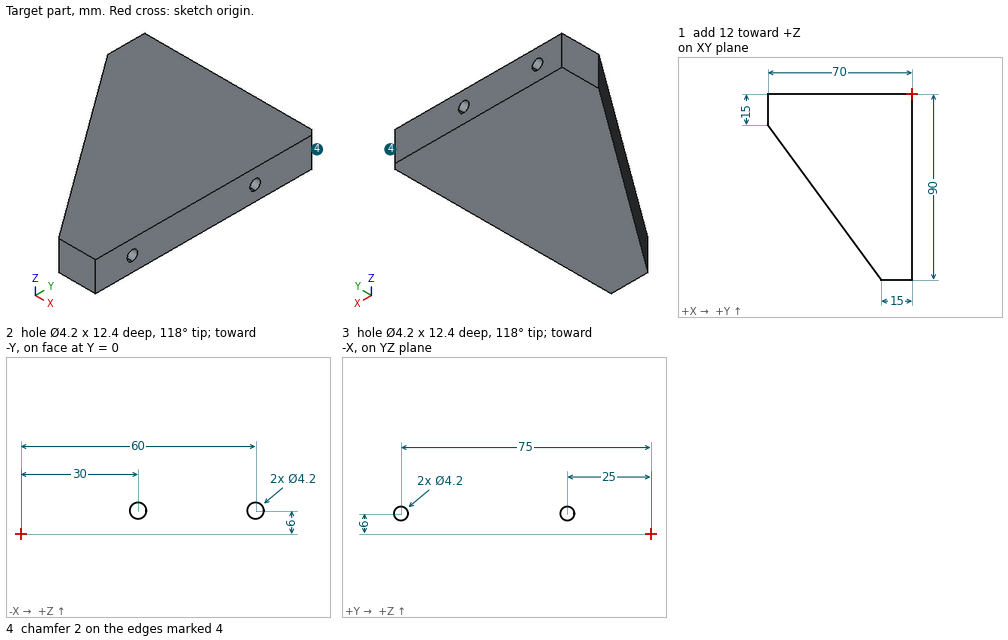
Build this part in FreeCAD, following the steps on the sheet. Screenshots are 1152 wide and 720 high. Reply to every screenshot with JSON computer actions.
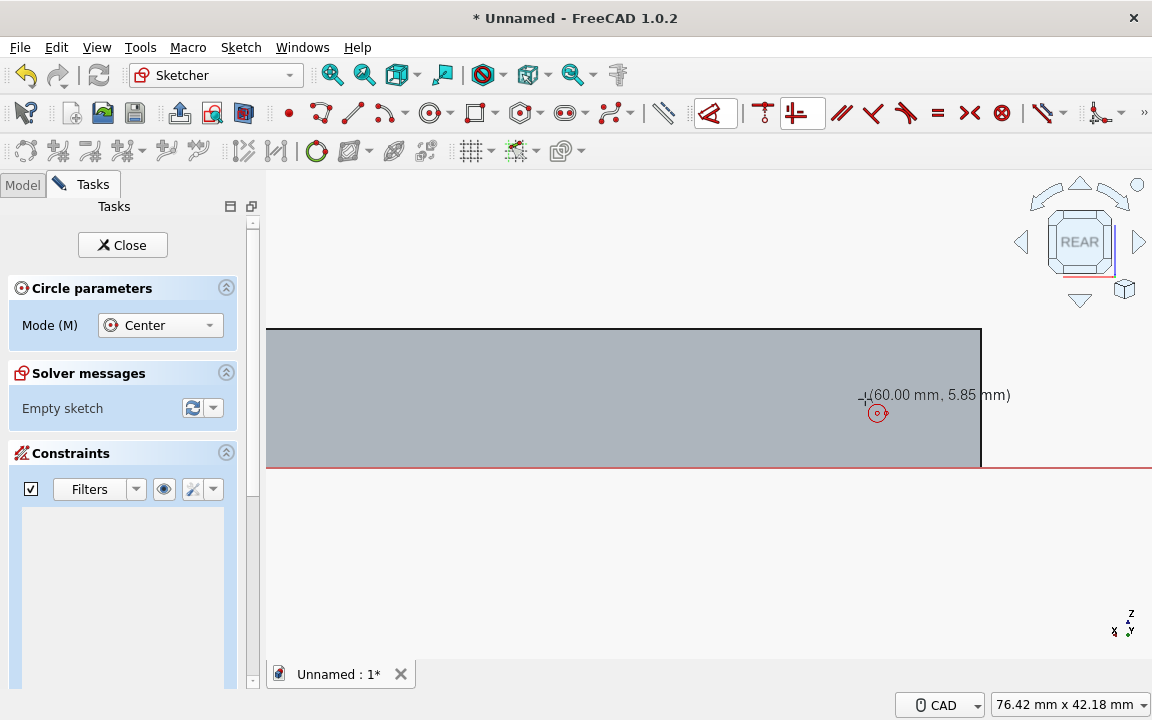
{"action": "left_click", "coordinate": [865, 399]}
{"action": "left_click", "coordinate": [882, 381]}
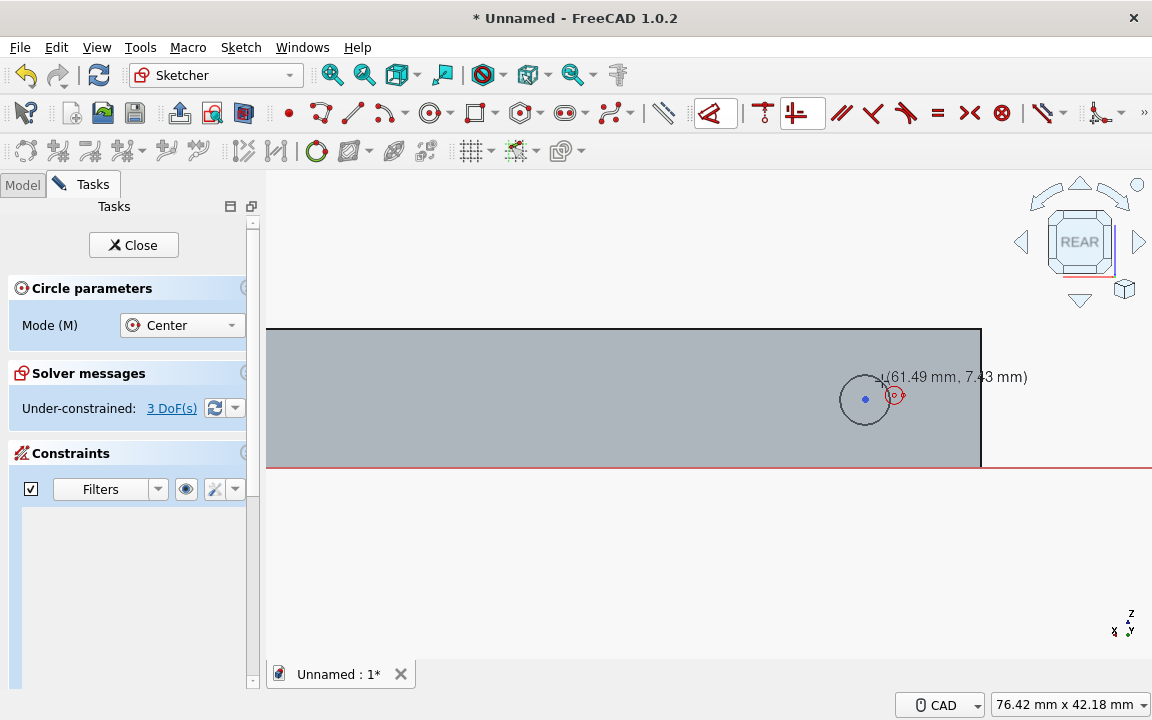
{"action": "left_click", "coordinate": [517, 399]}
{"action": "left_click", "coordinate": [534, 381]}
{"action": "key", "text": "Escape"}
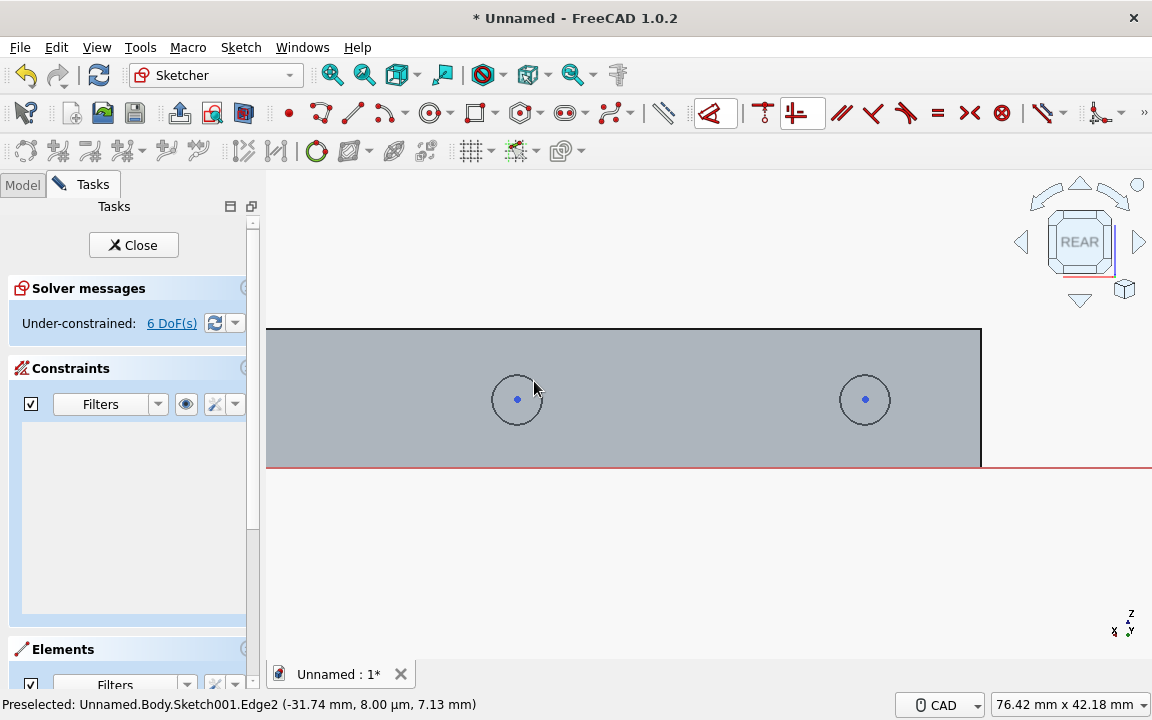
{"action": "left_click", "coordinate": [882, 382]}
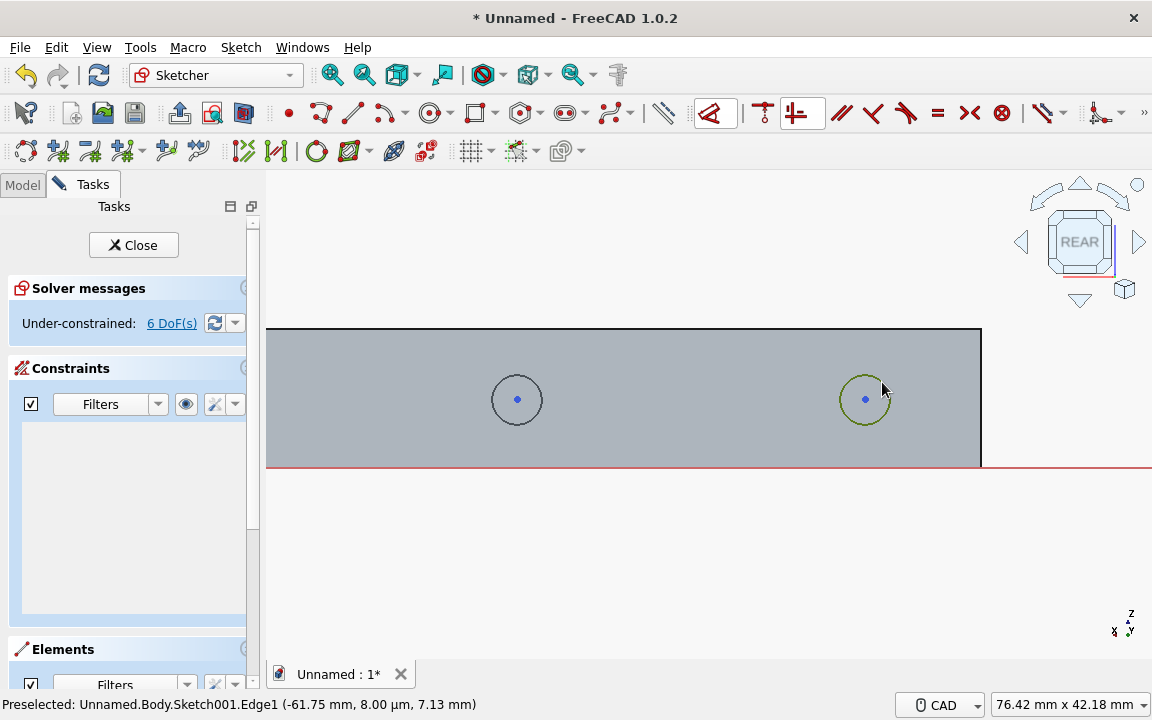
{"action": "left_click", "coordinate": [534, 382]}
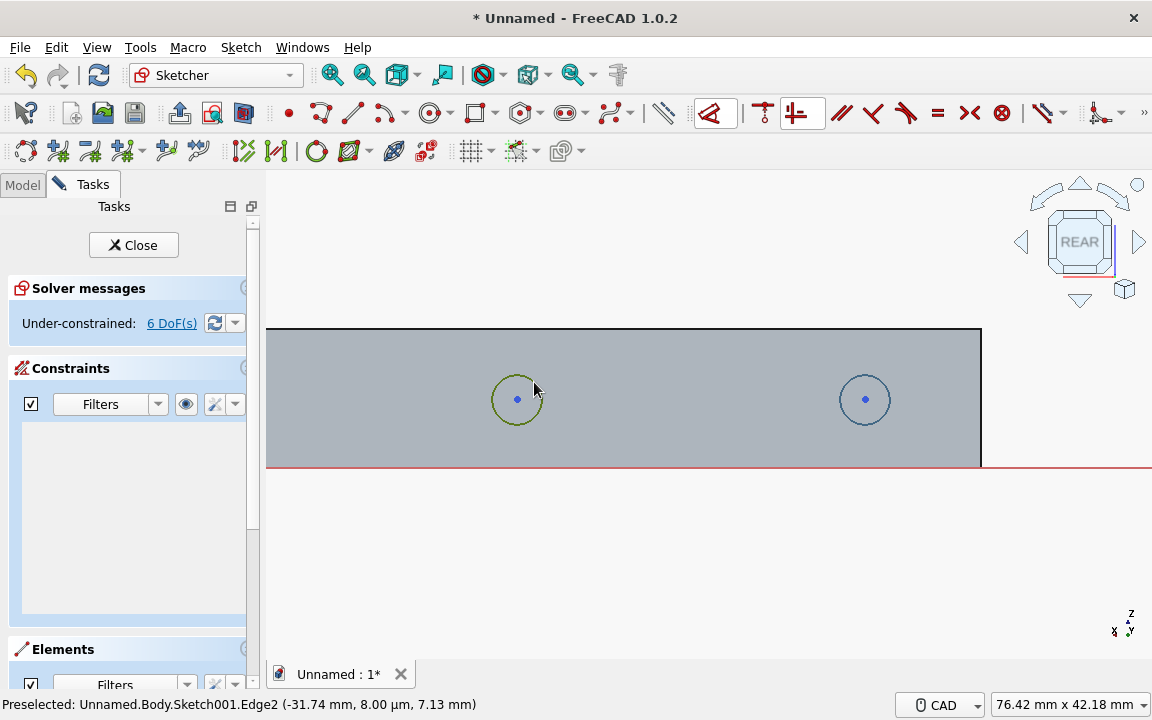
{"action": "key", "text": "e"}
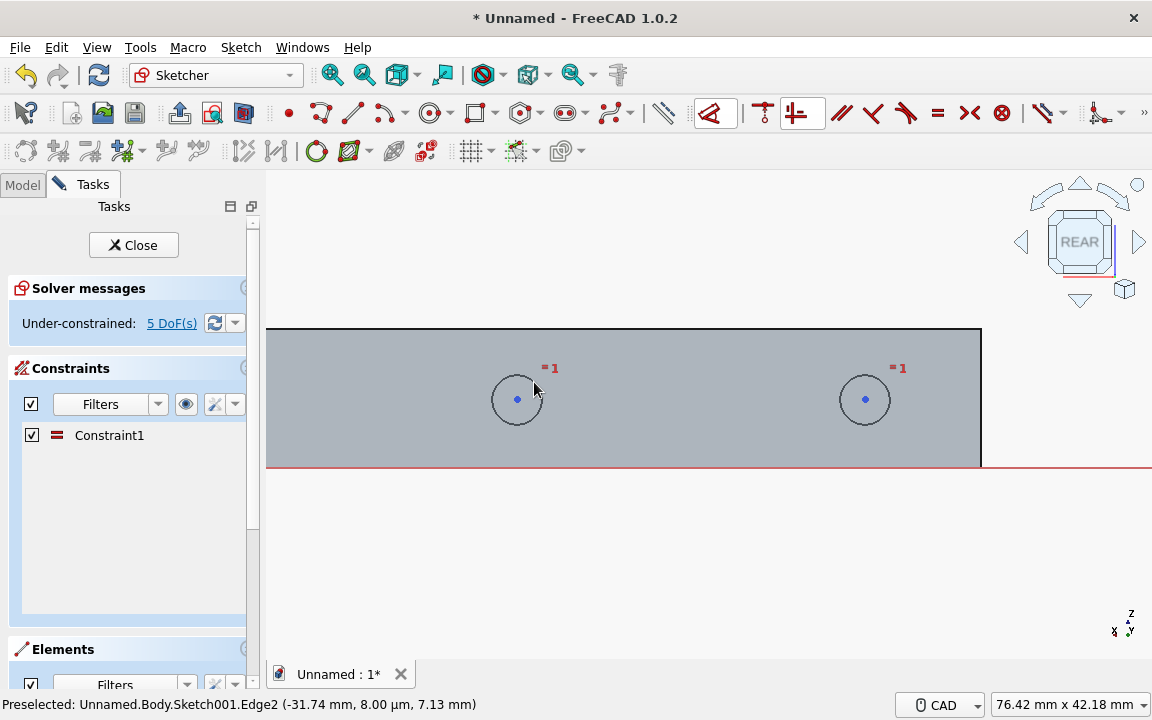
{"action": "left_click", "coordinate": [865, 400]}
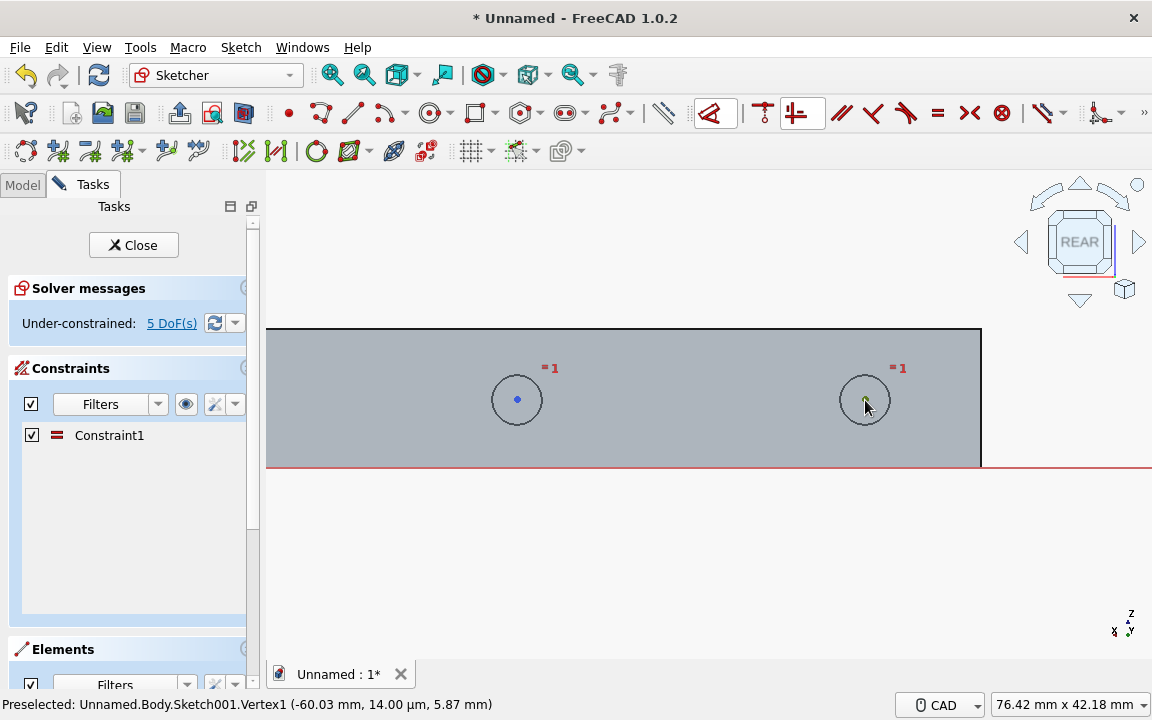
{"action": "left_click", "coordinate": [517, 400]}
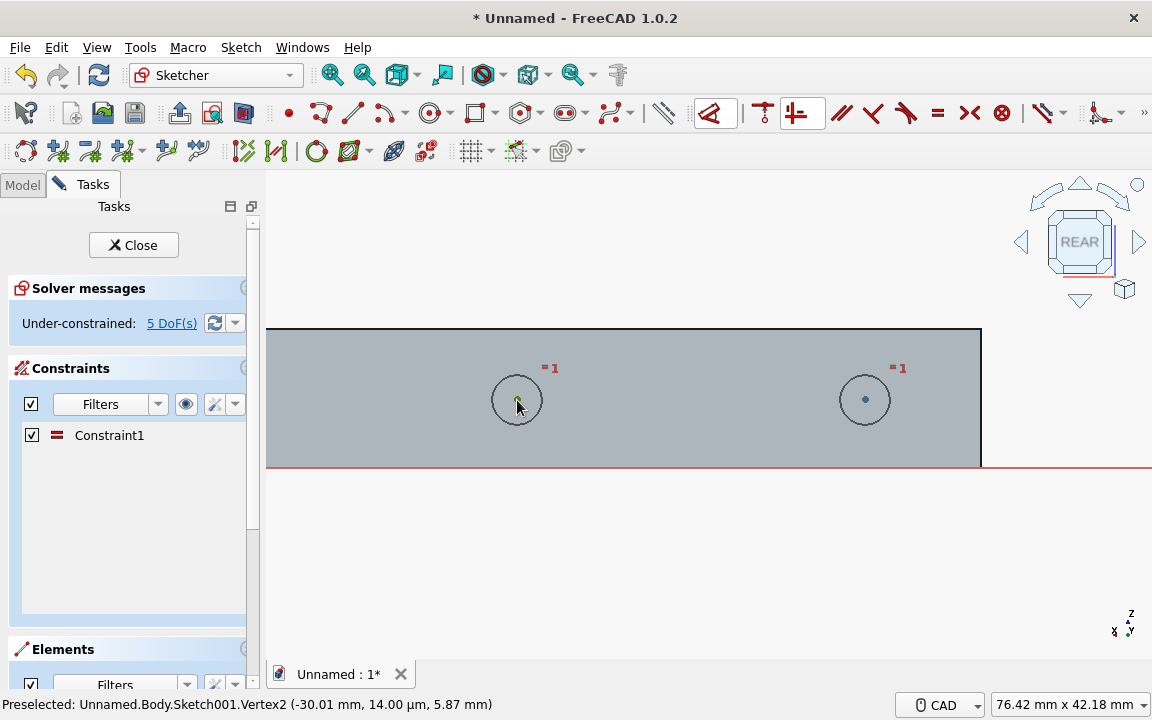
{"action": "left_click", "coordinate": [820, 114]}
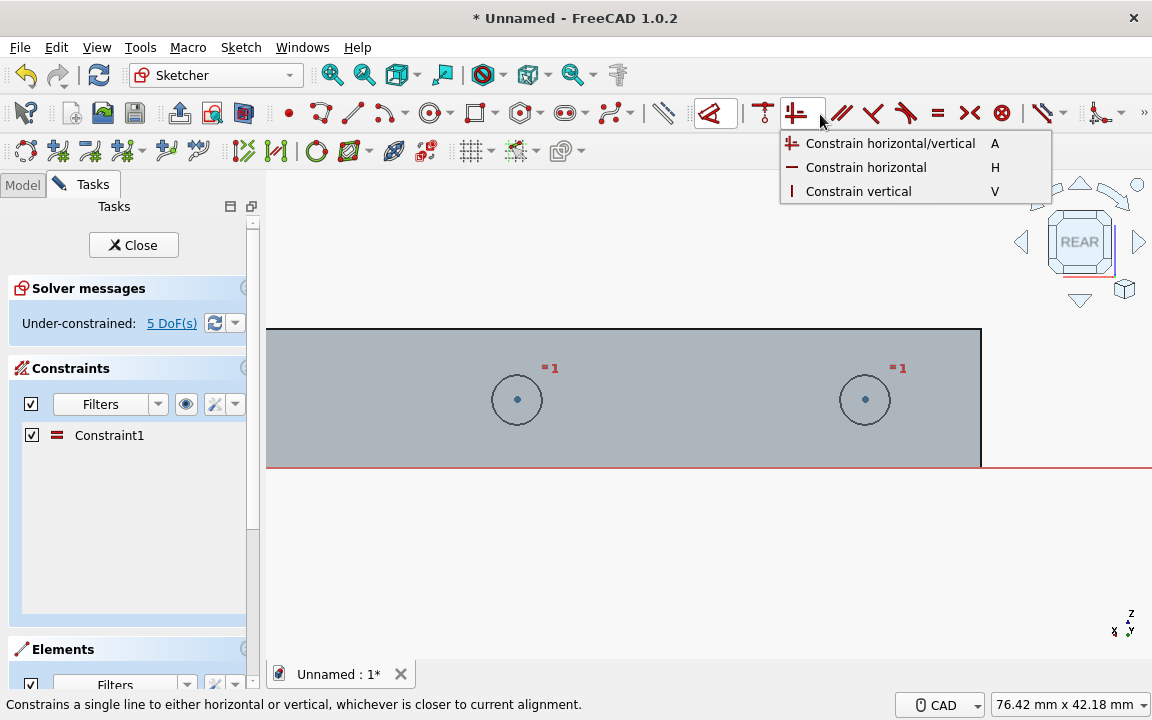
{"action": "left_click", "coordinate": [916, 167]}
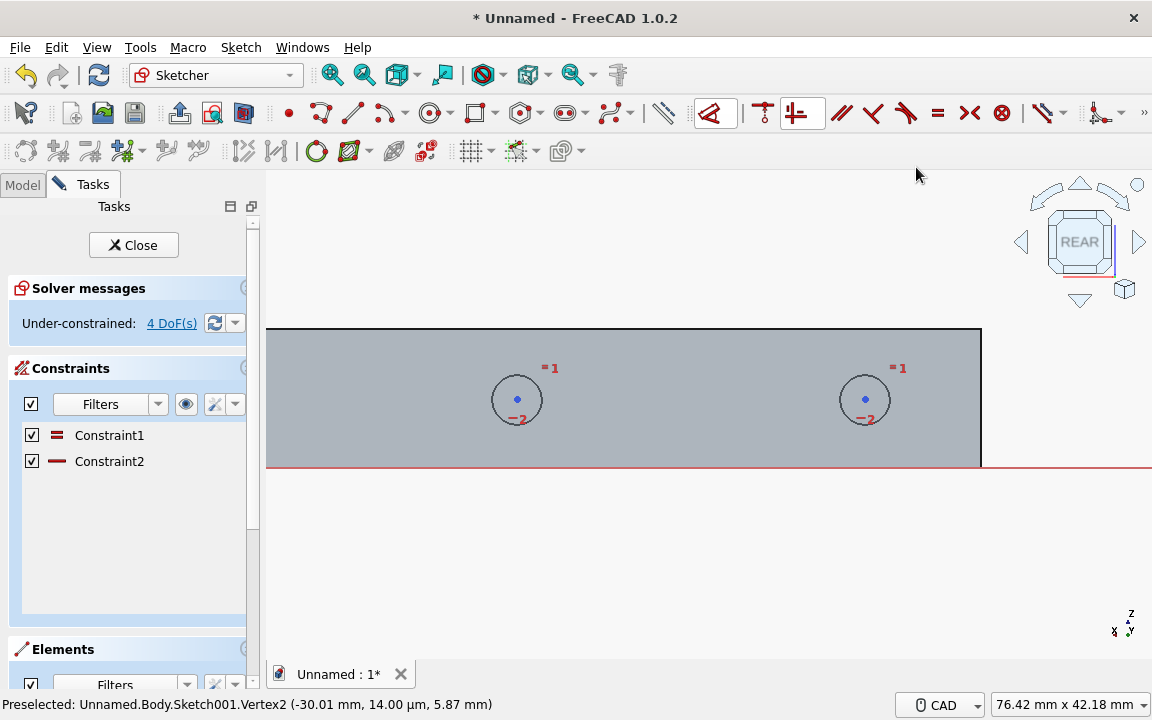
{"action": "left_click", "coordinate": [882, 382]}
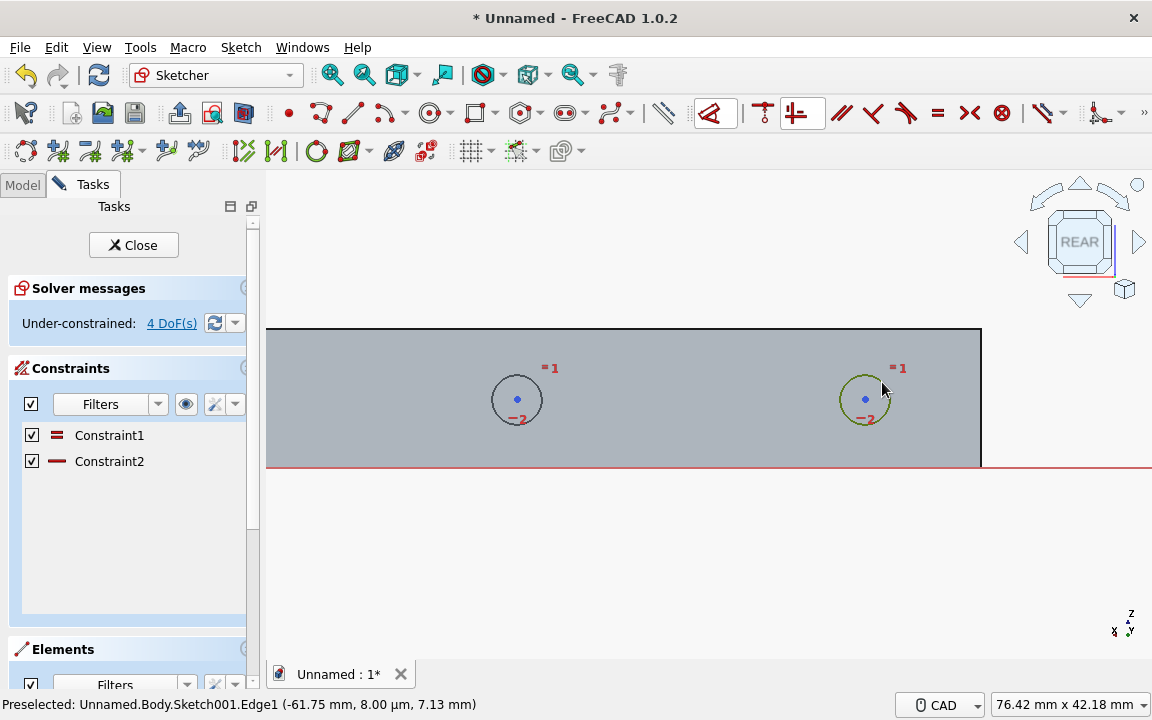
{"action": "left_click", "coordinate": [732, 114]}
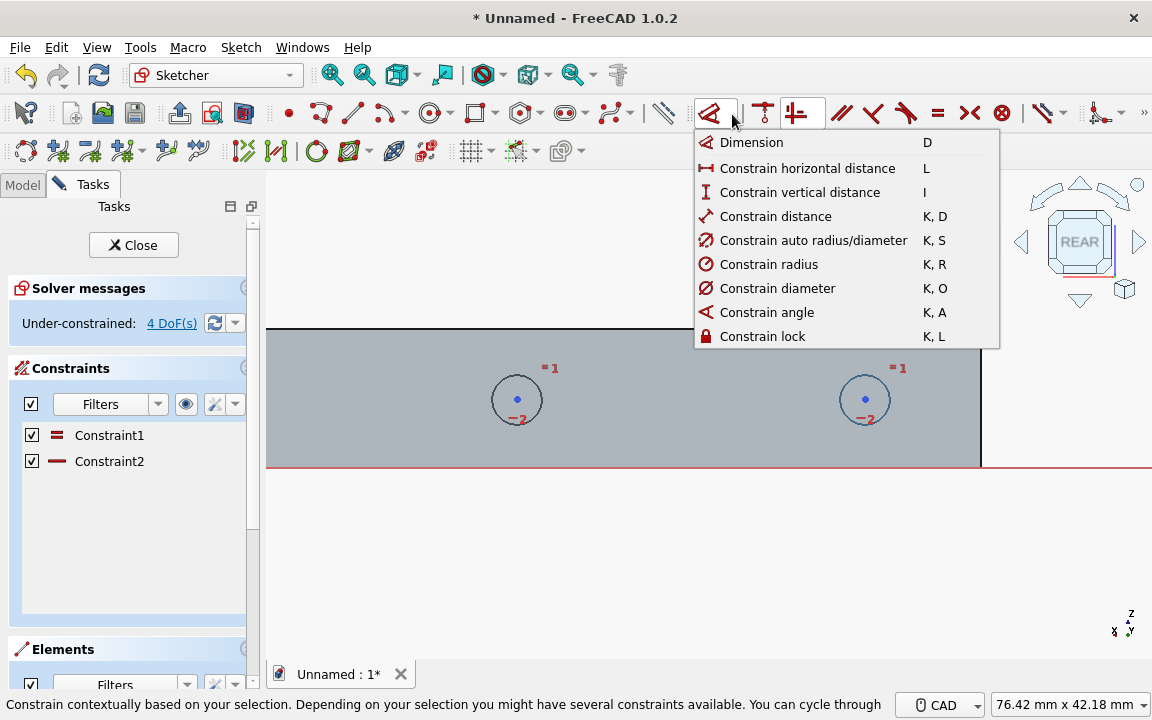
{"action": "left_click", "coordinate": [847, 288]}